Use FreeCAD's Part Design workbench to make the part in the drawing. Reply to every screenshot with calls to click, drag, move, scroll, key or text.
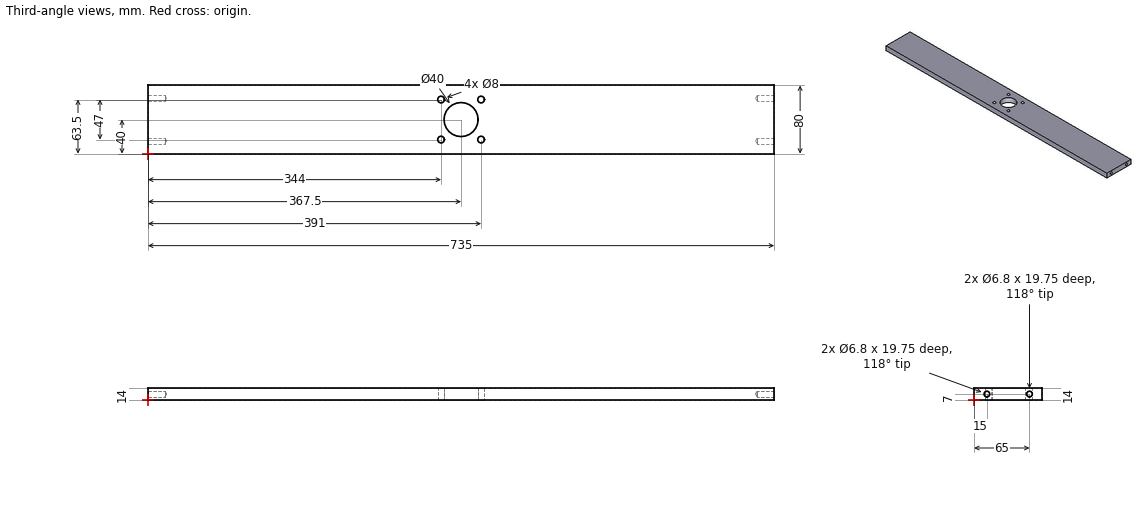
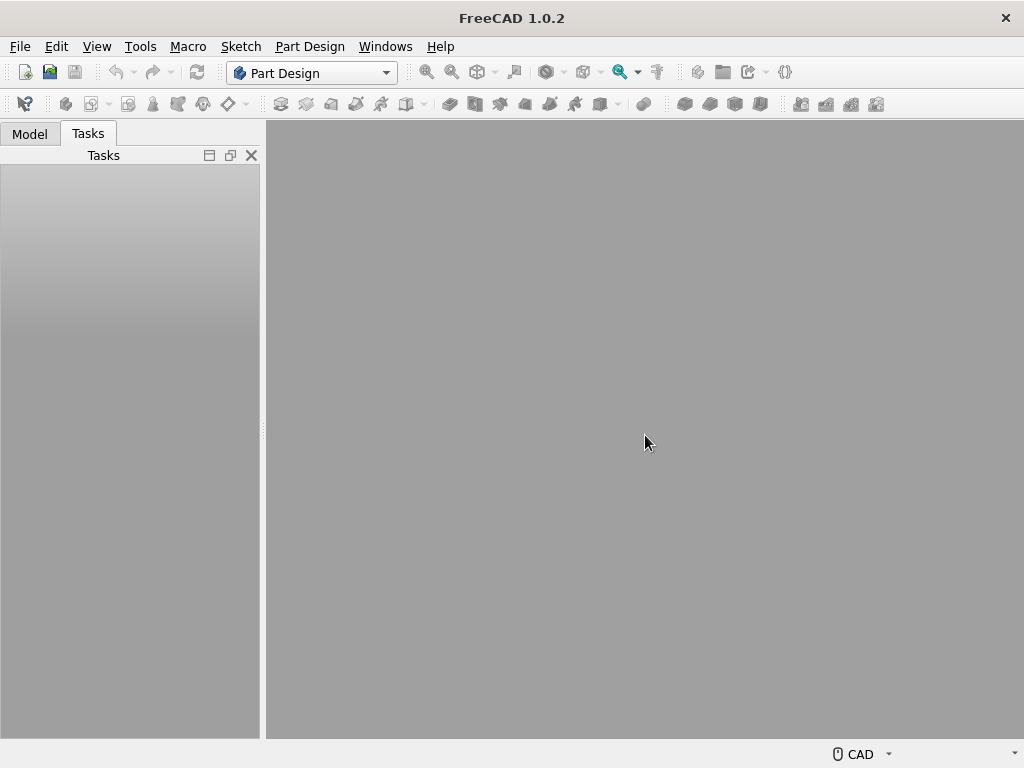
click(25, 72)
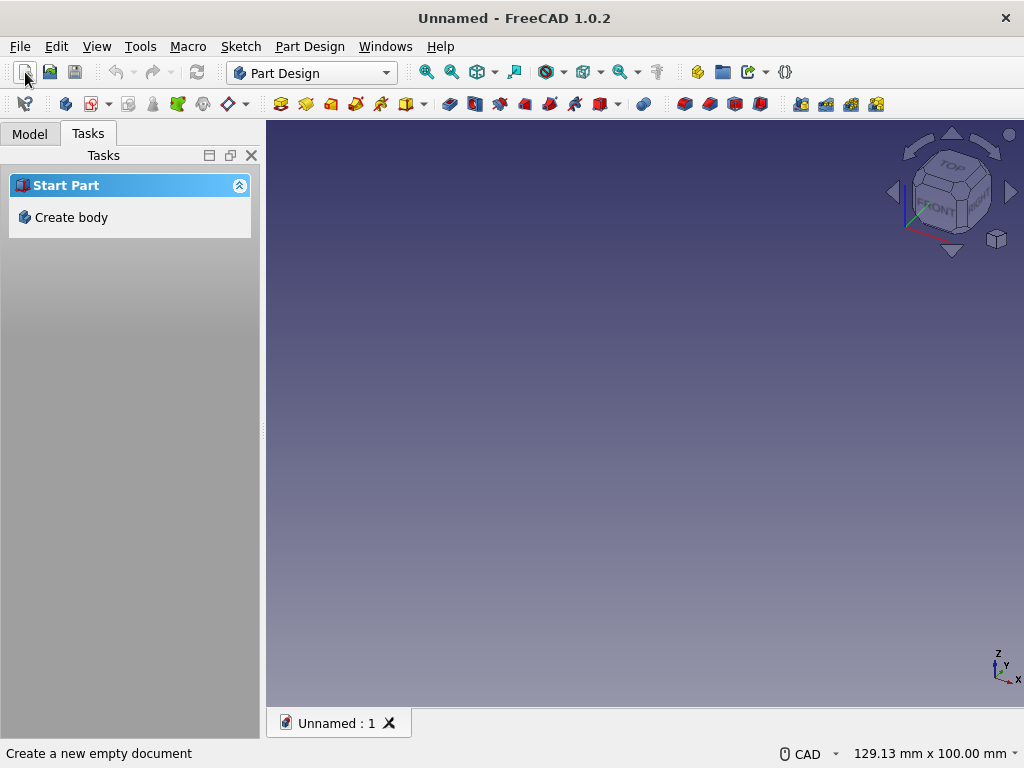
click(90, 104)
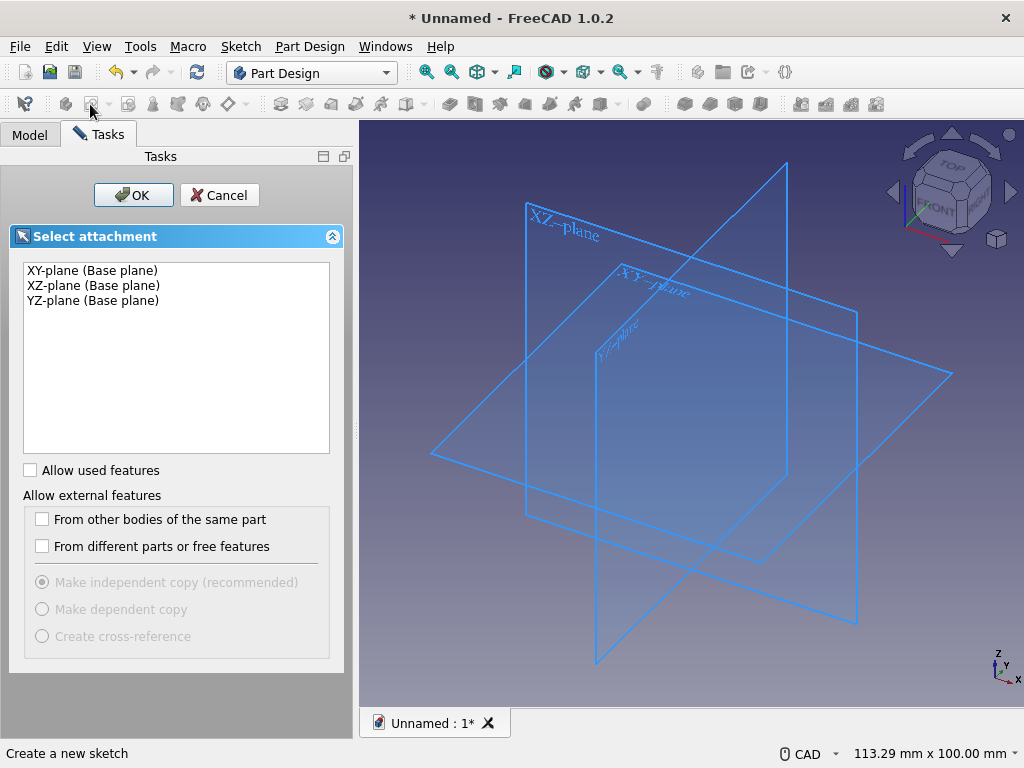
click(84, 270)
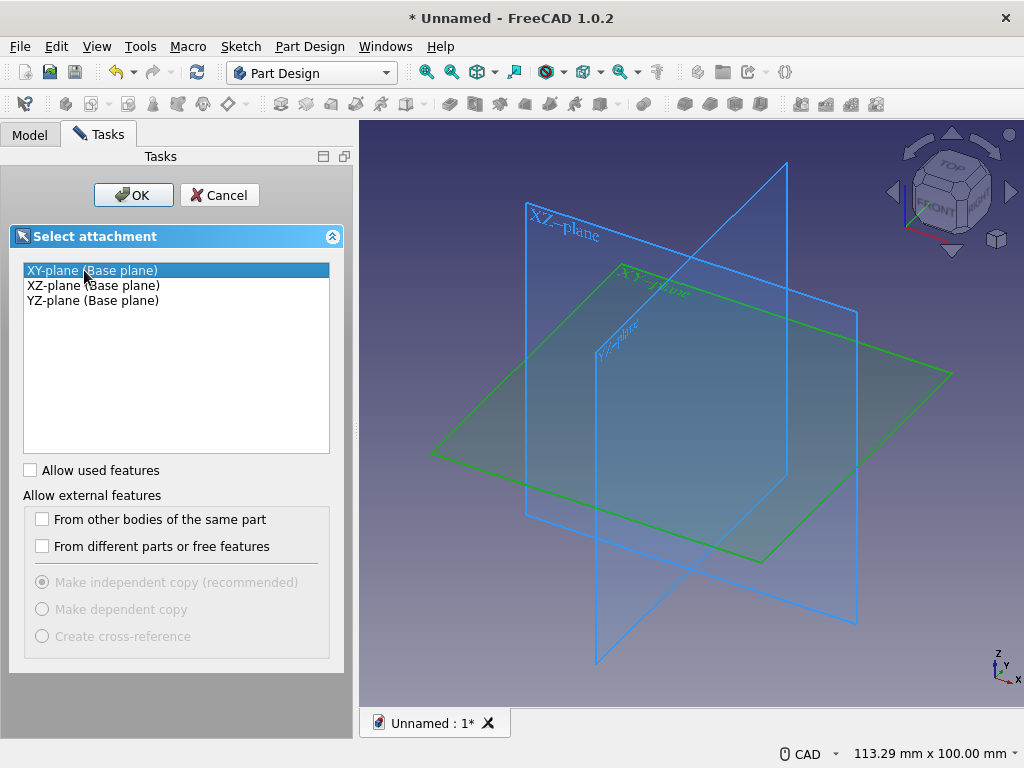
click(134, 195)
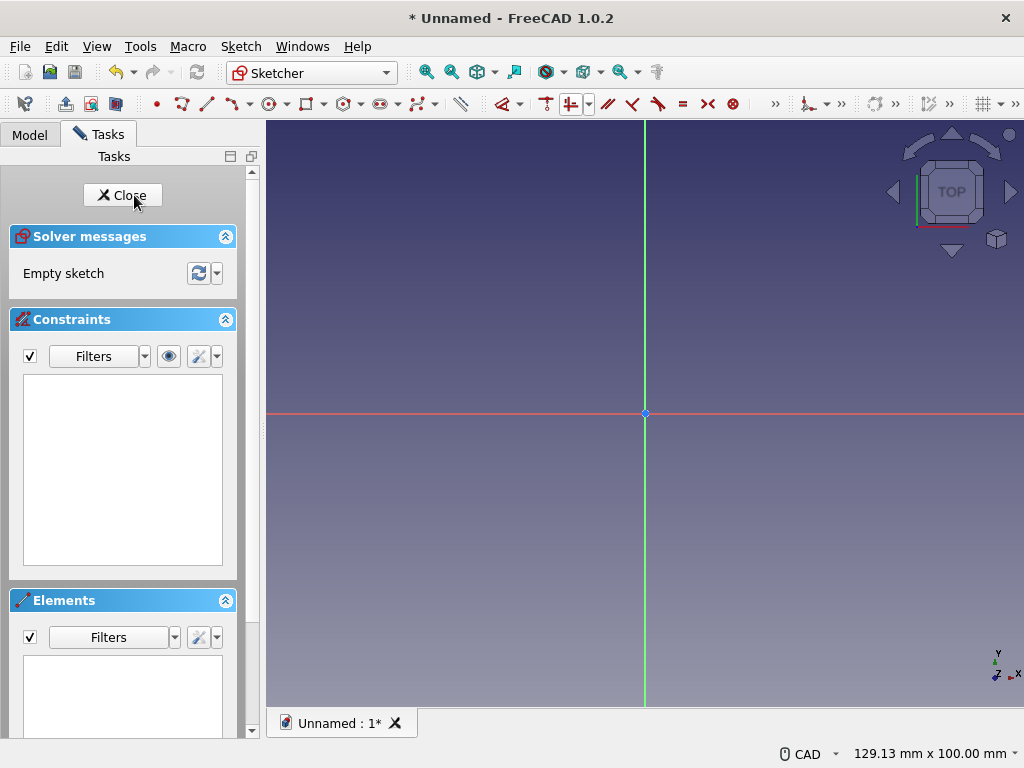
scroll(354, 437, down, 12)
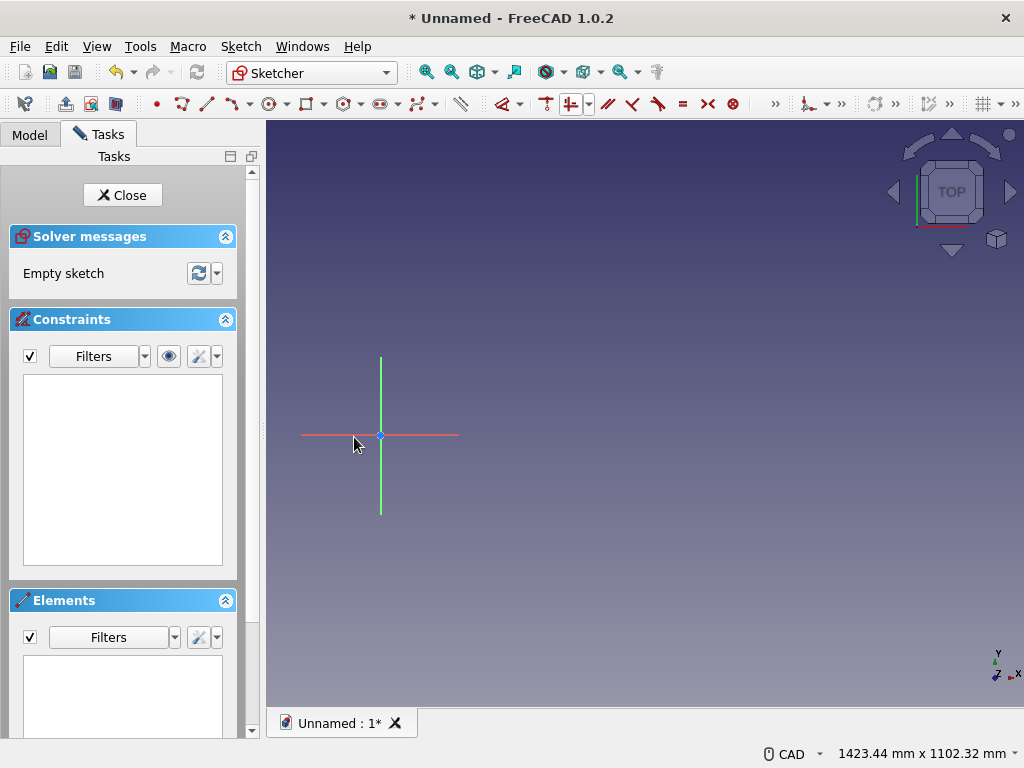
key(g)
key(r)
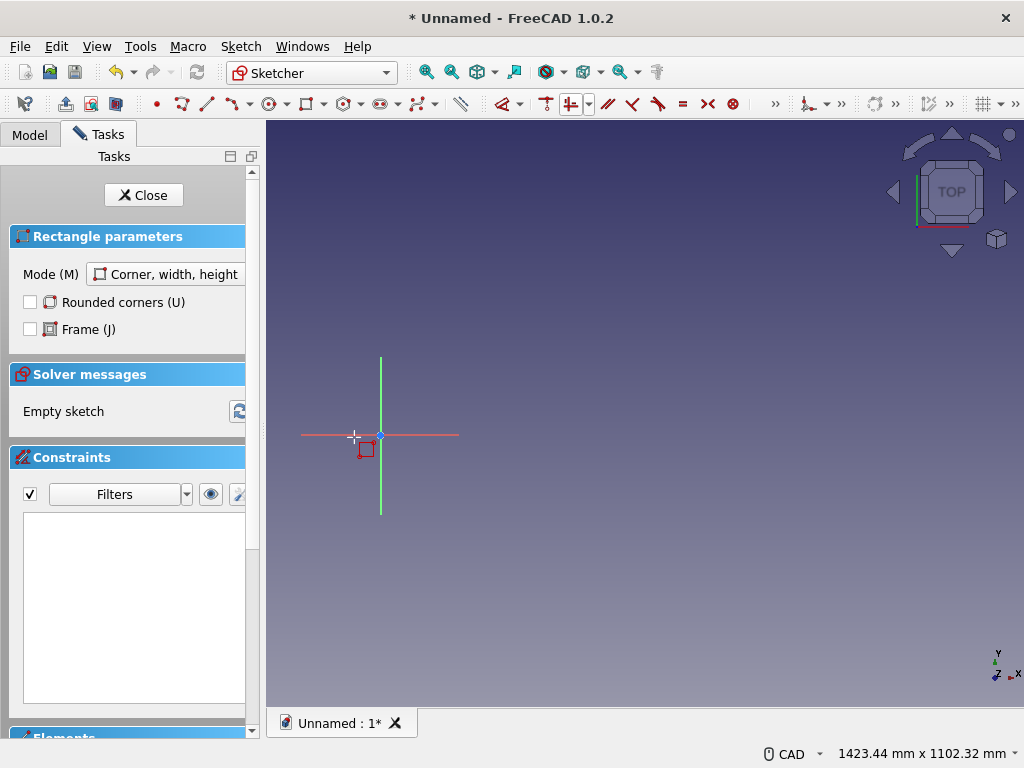
click(381, 435)
move(772, 393)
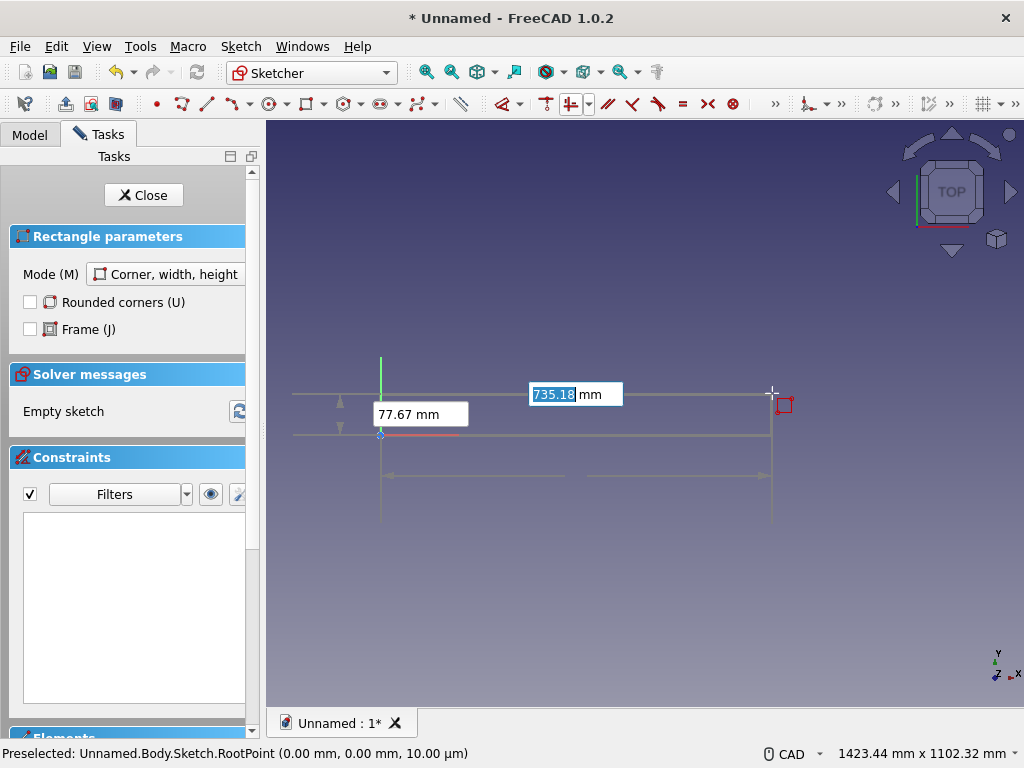
text(735)
key(Tab)
text(80)
key(Return)
key(Escape)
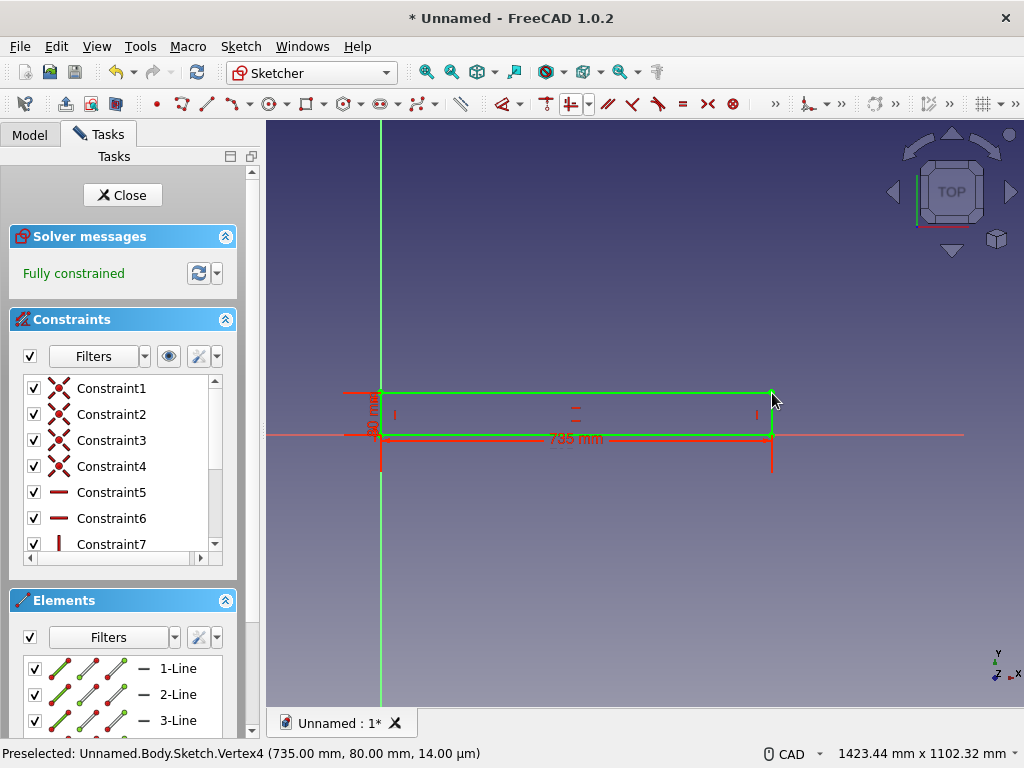
click(123, 195)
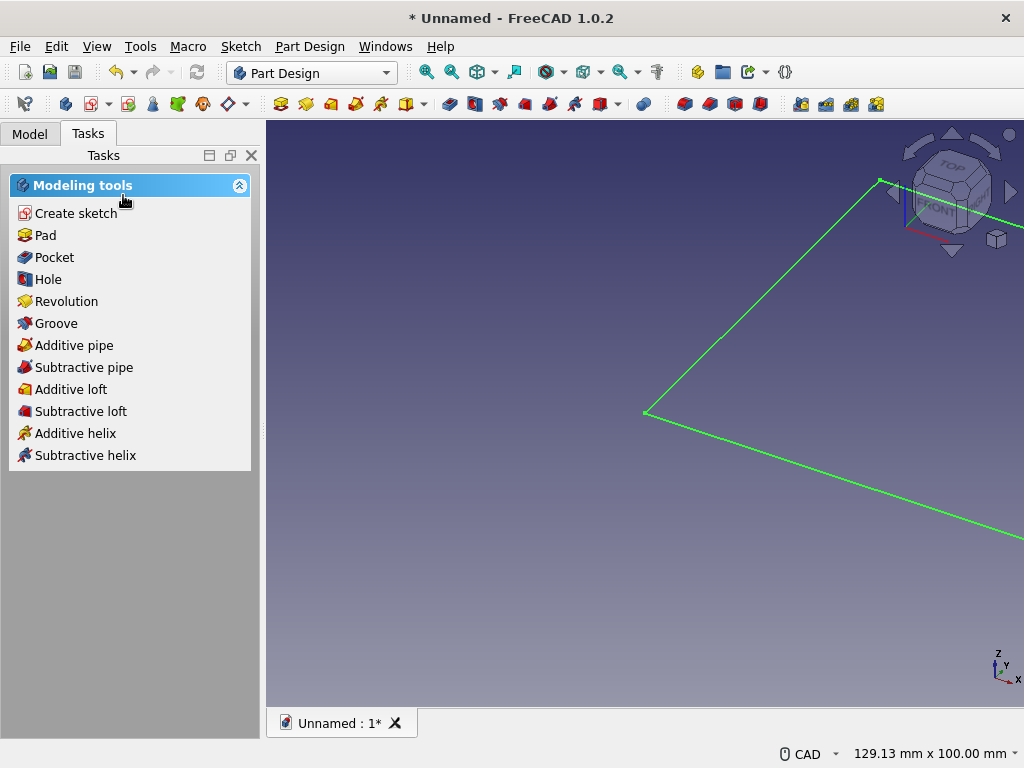
click(281, 104)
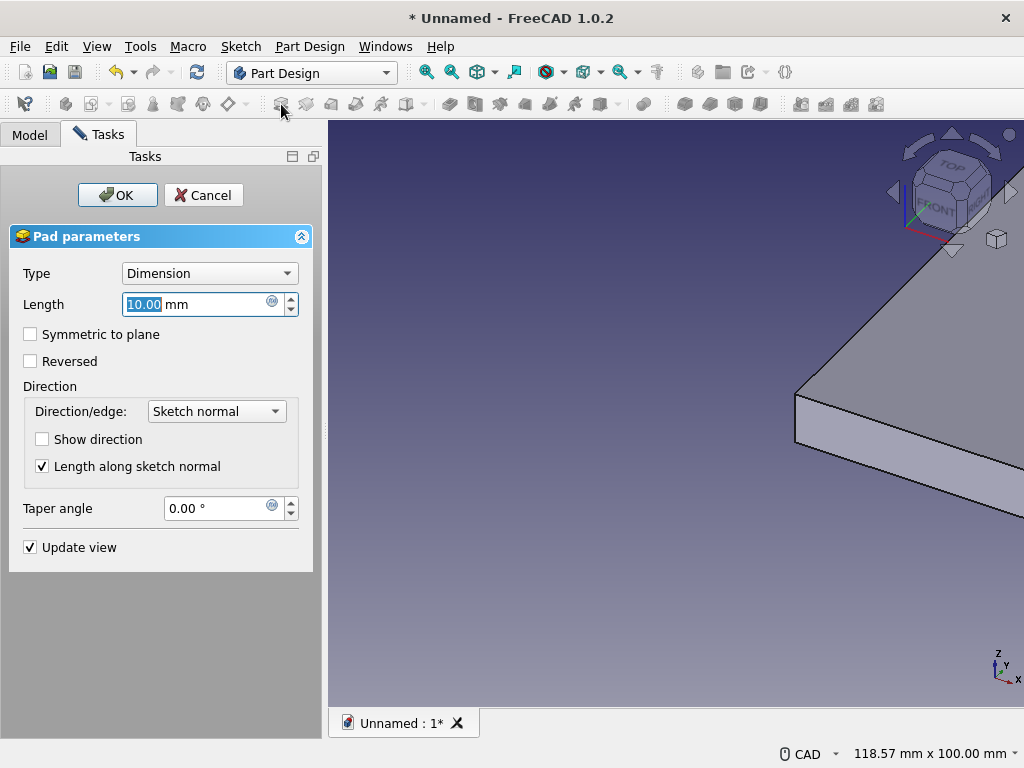
text(14)
key(Tab)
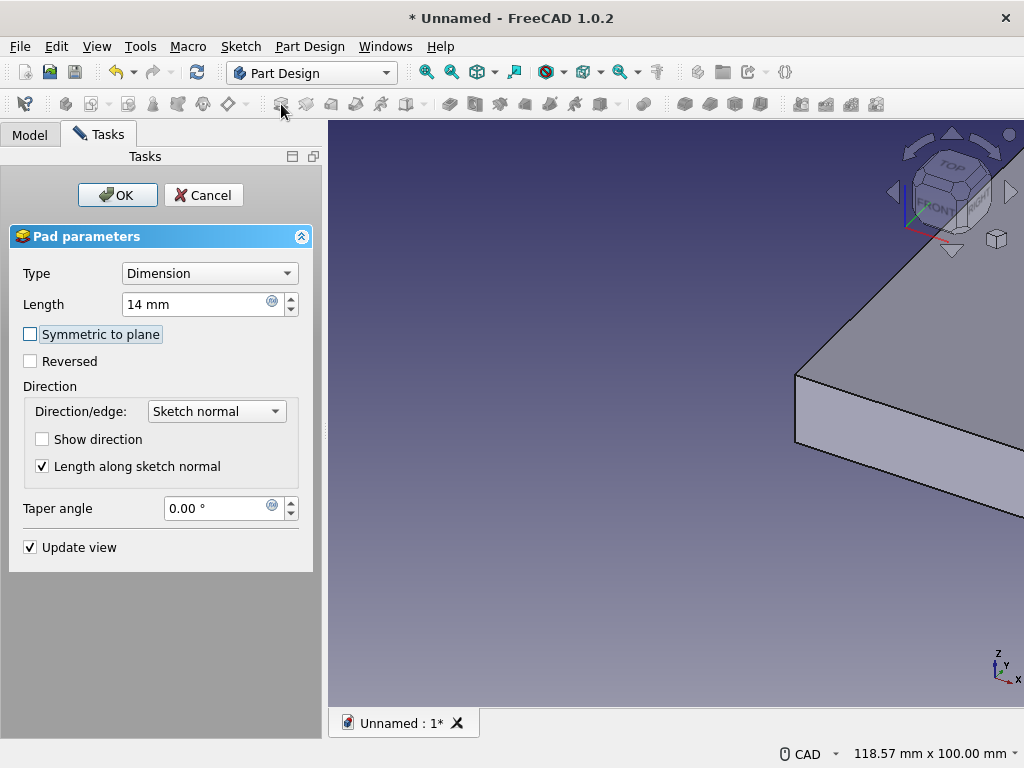
click(118, 195)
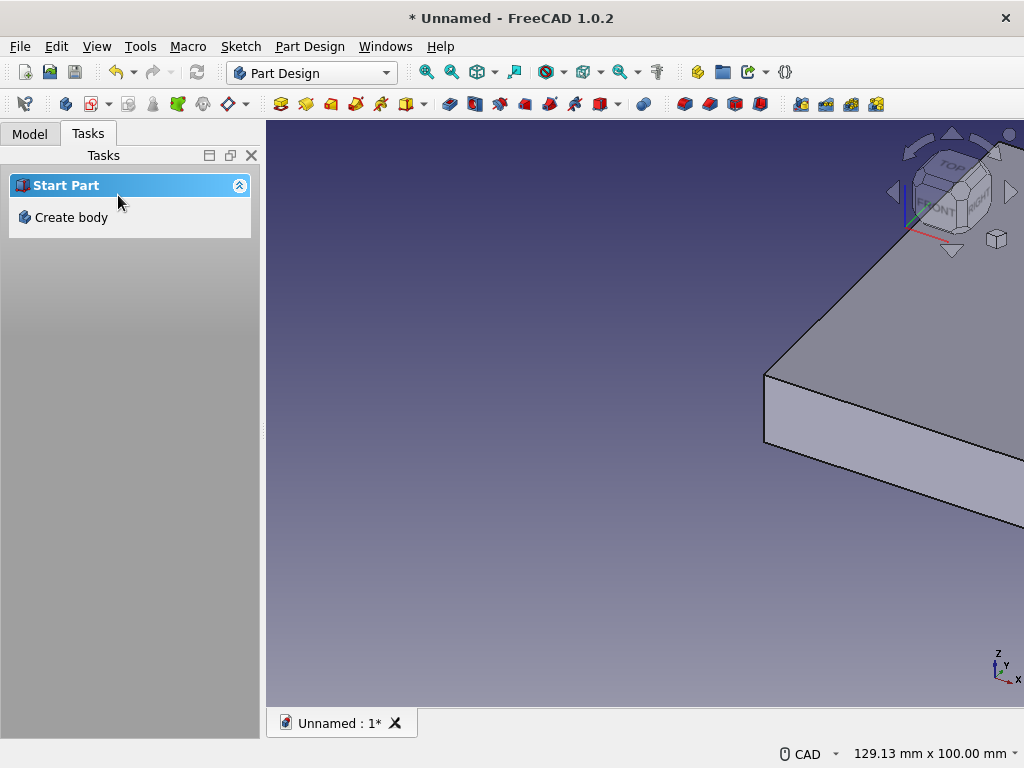
click(427, 72)